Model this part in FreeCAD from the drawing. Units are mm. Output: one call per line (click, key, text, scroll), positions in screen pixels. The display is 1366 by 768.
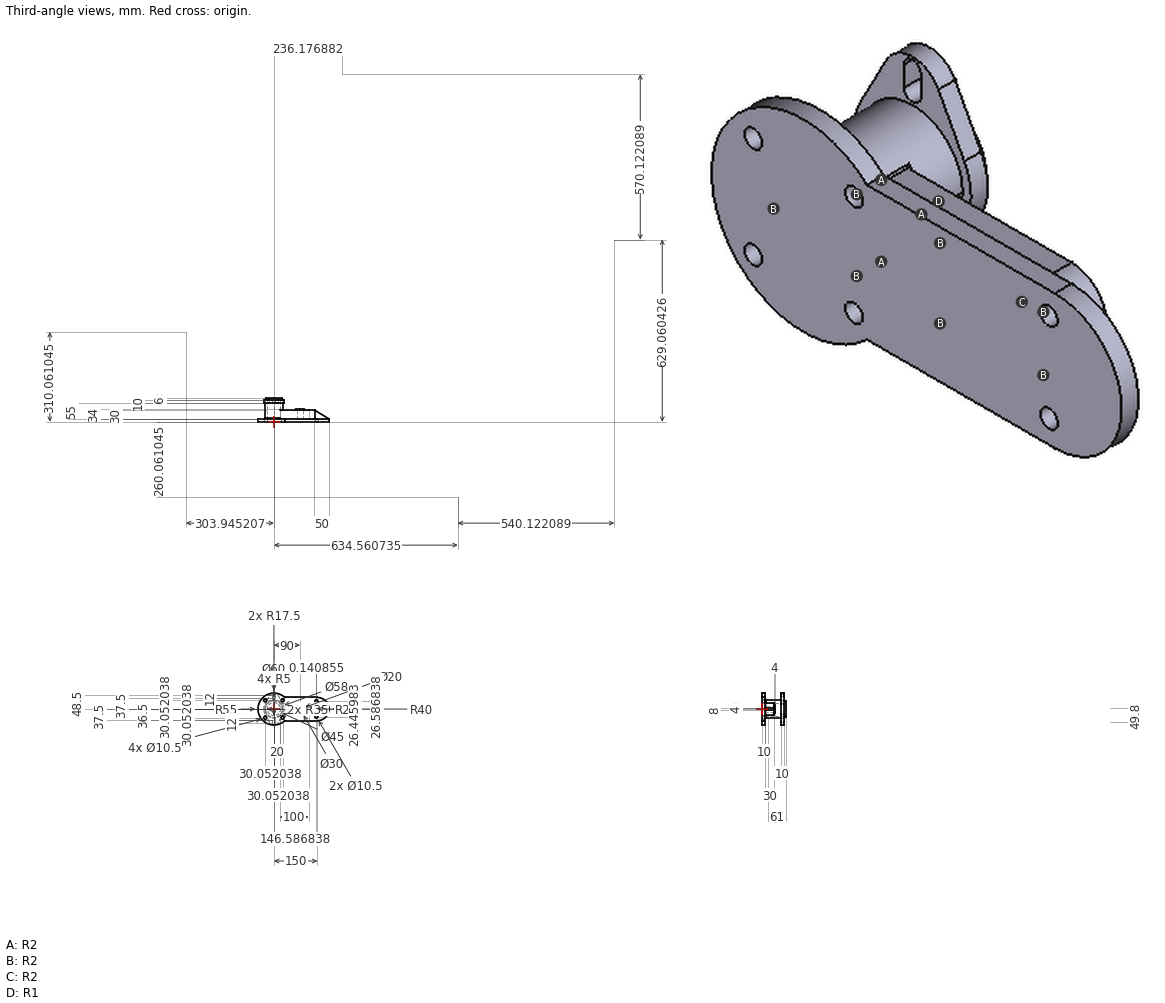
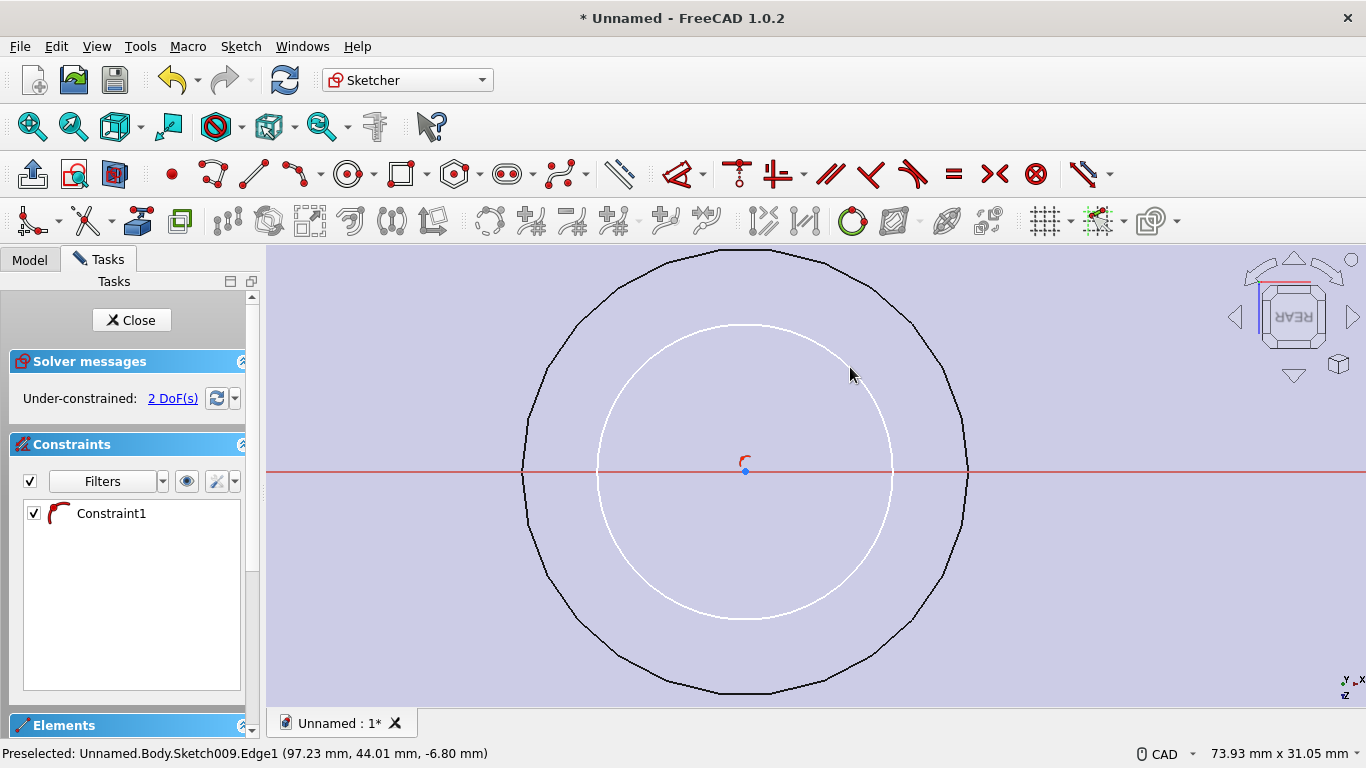
key(d)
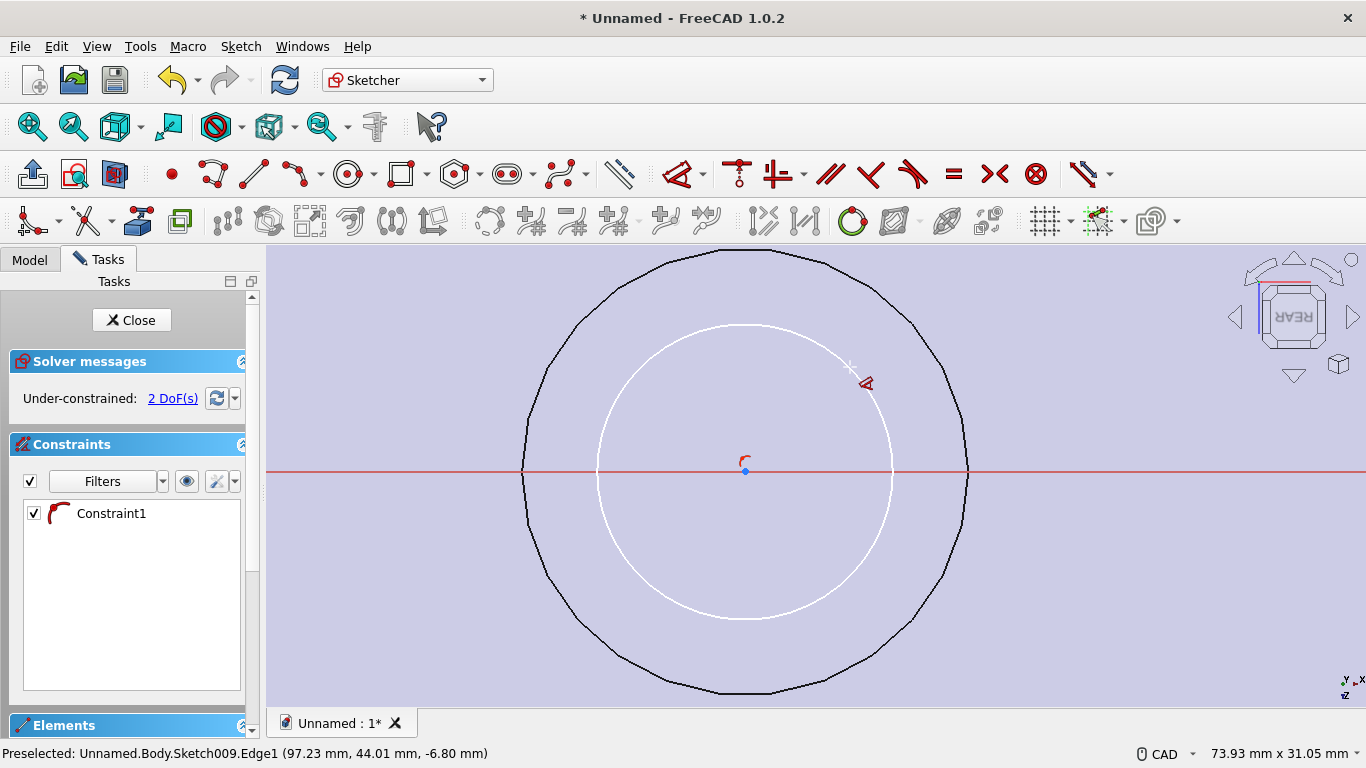
click(849, 367)
click(872, 344)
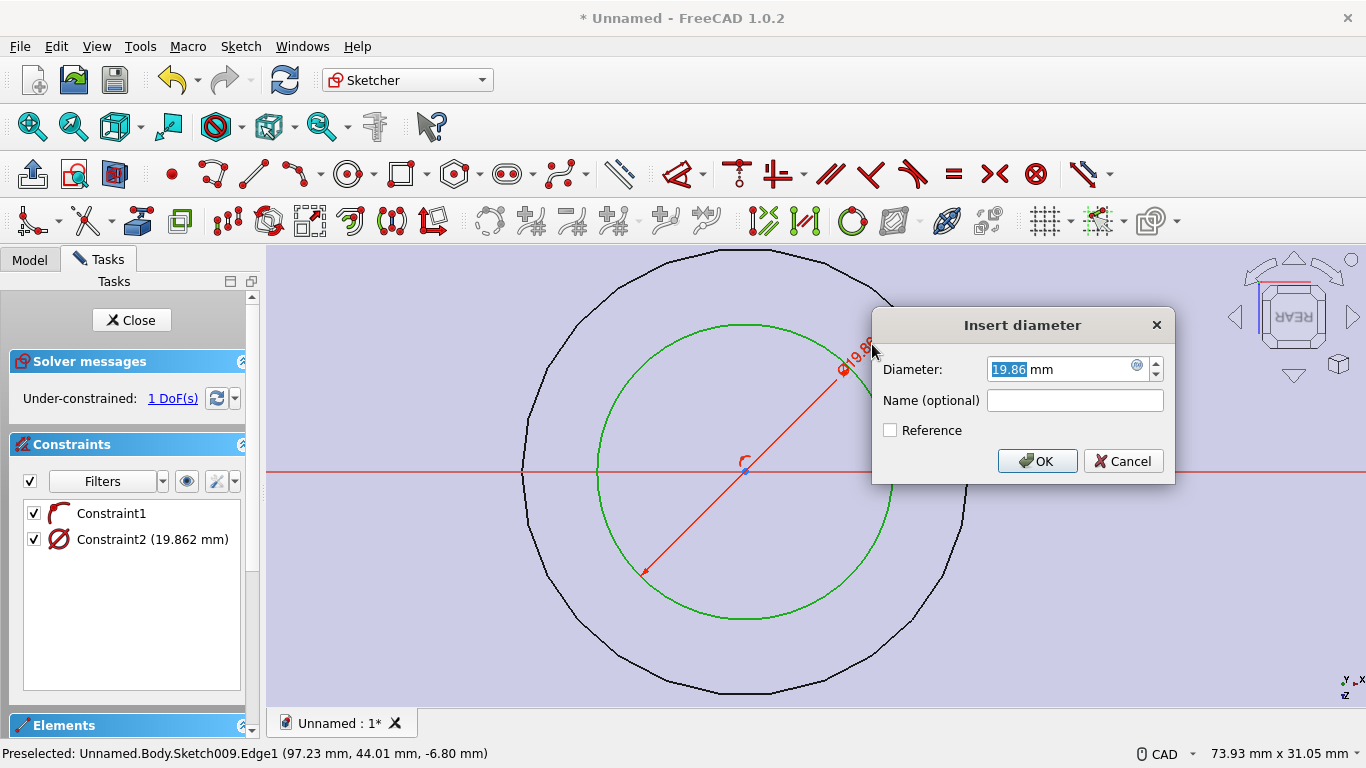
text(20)
key(Return)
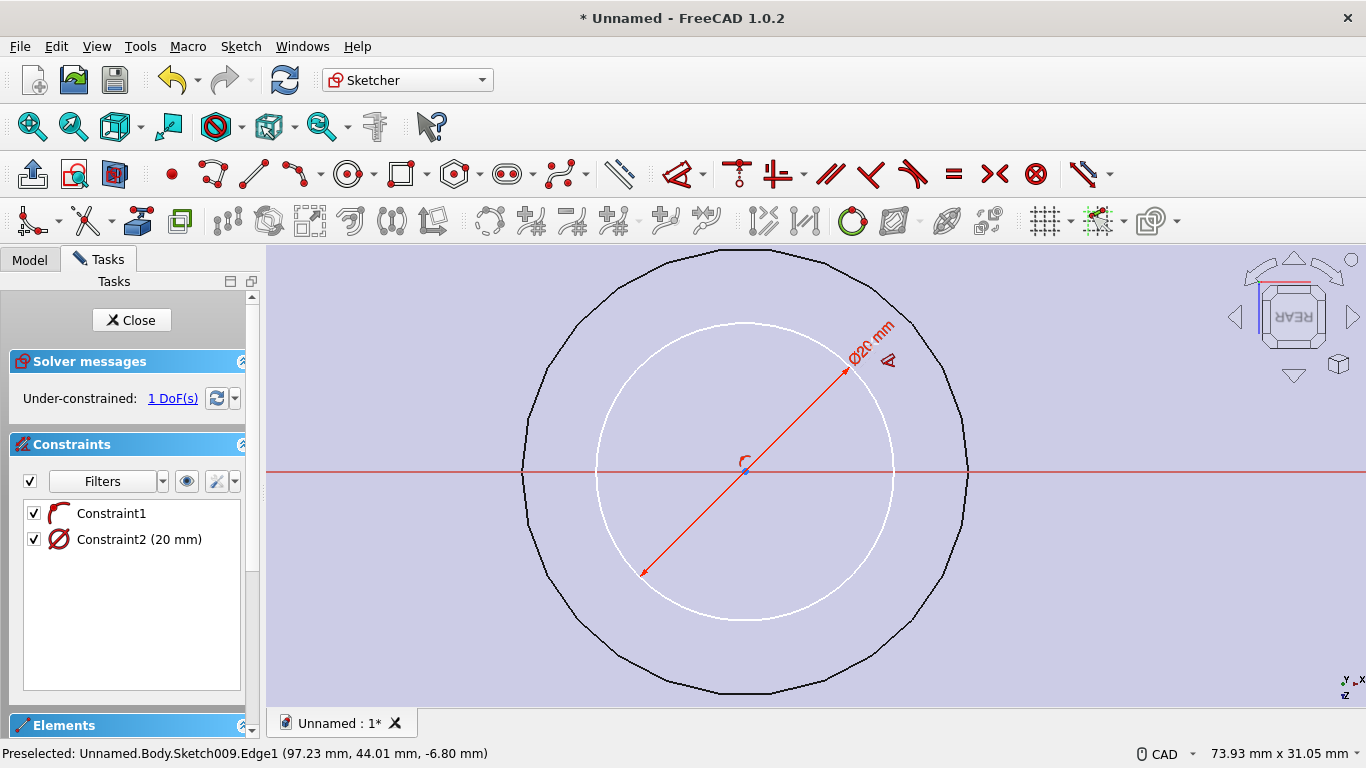
click(745, 472)
click(520, 506)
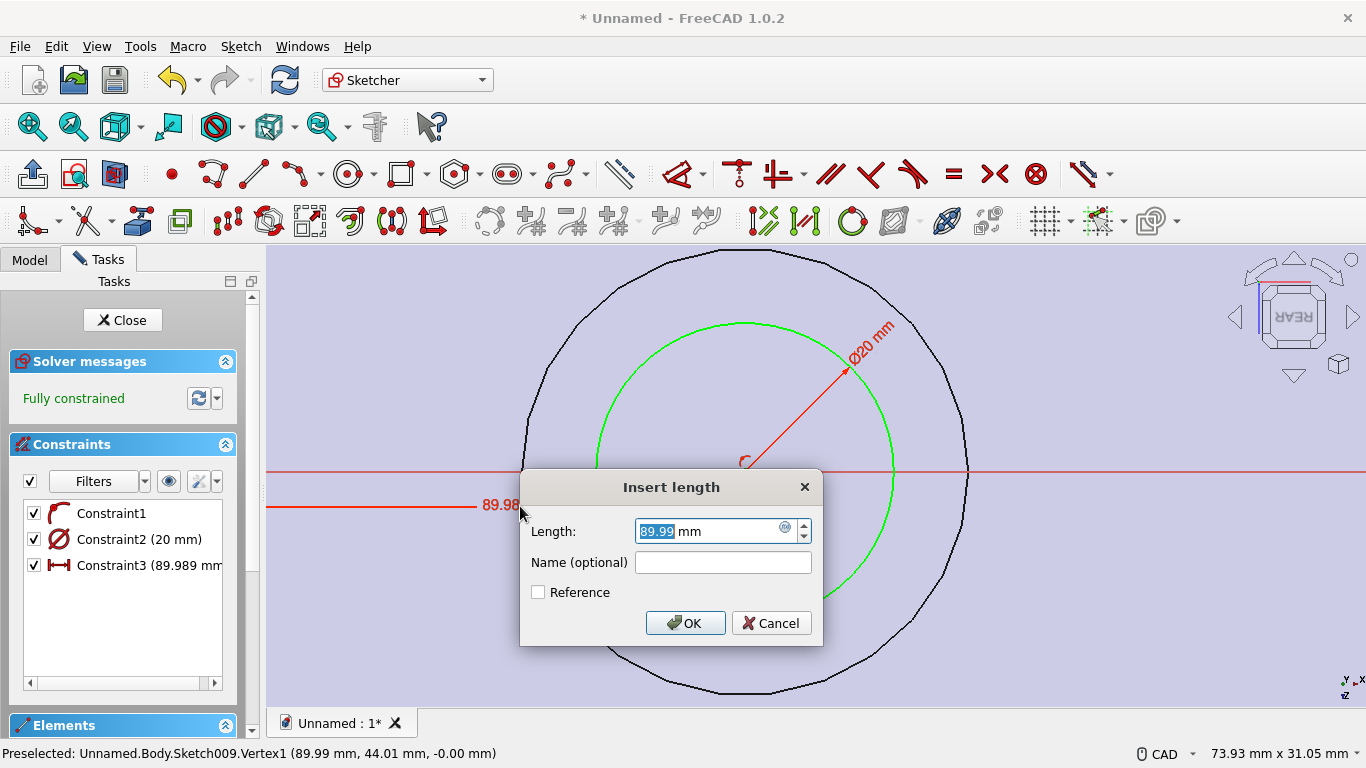
text(90)
key(Return)
key(Escape)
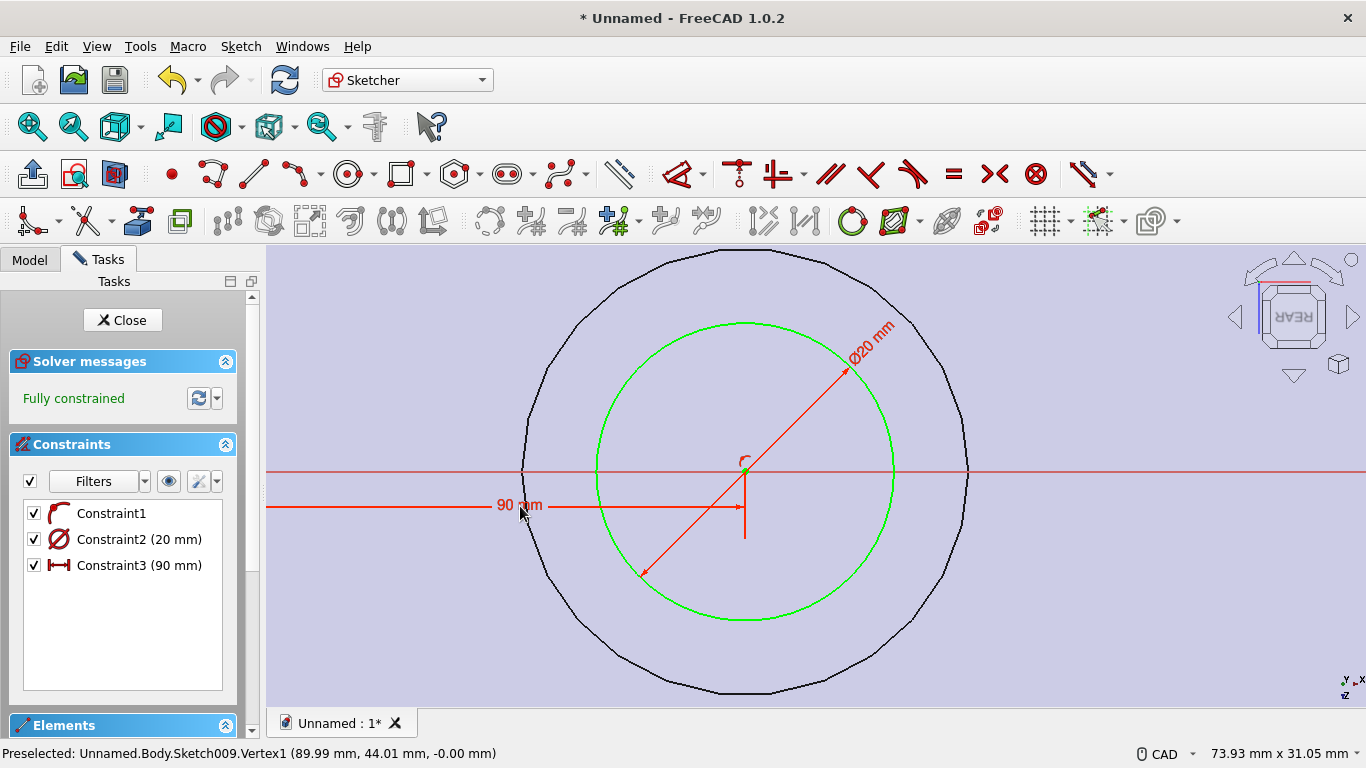
click(123, 320)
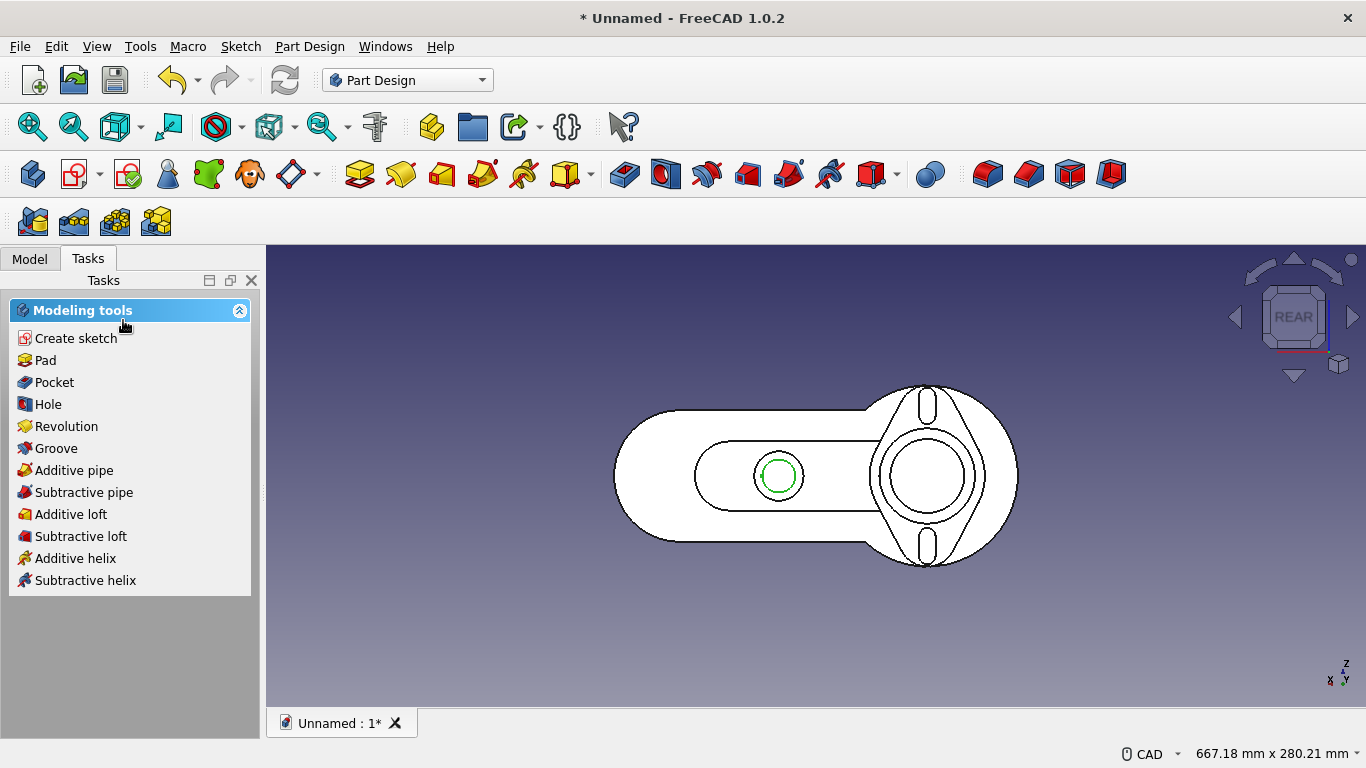
click(625, 174)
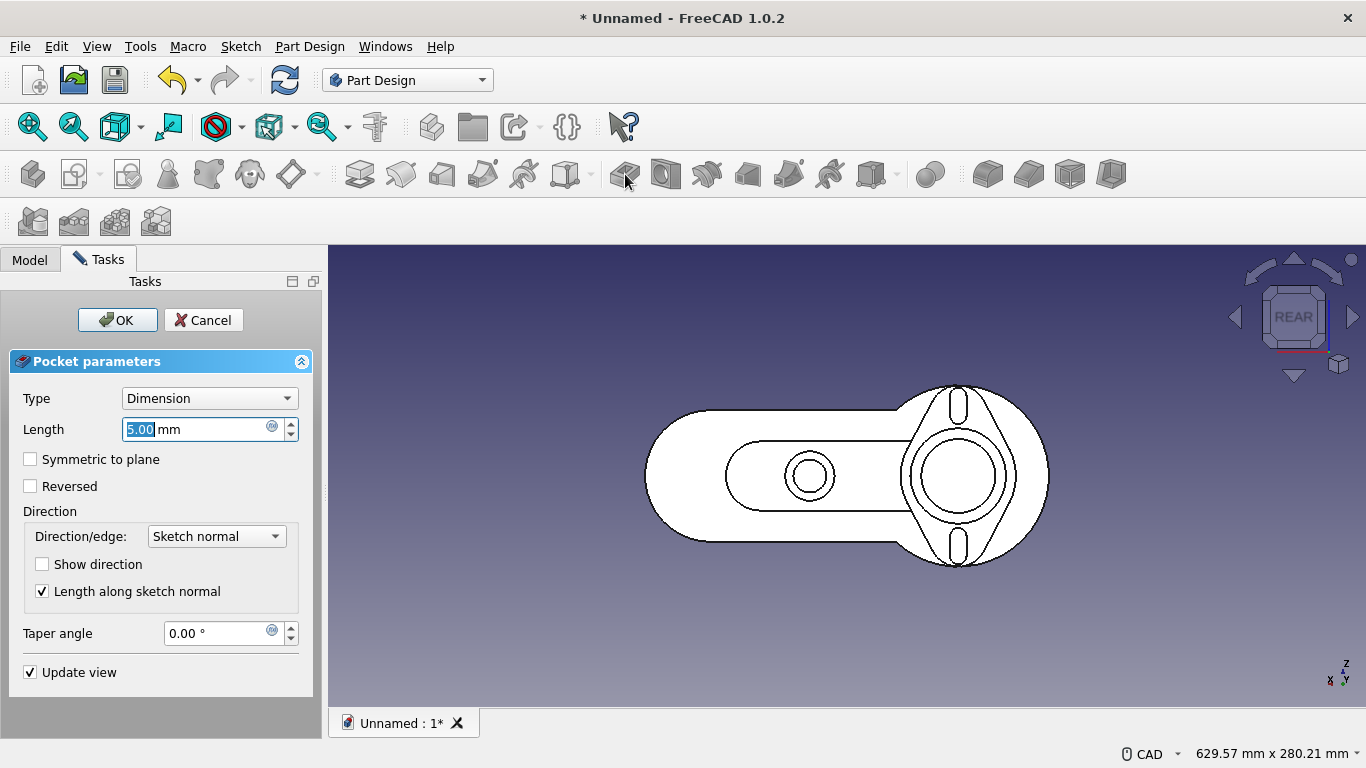
text(34)
key(Tab)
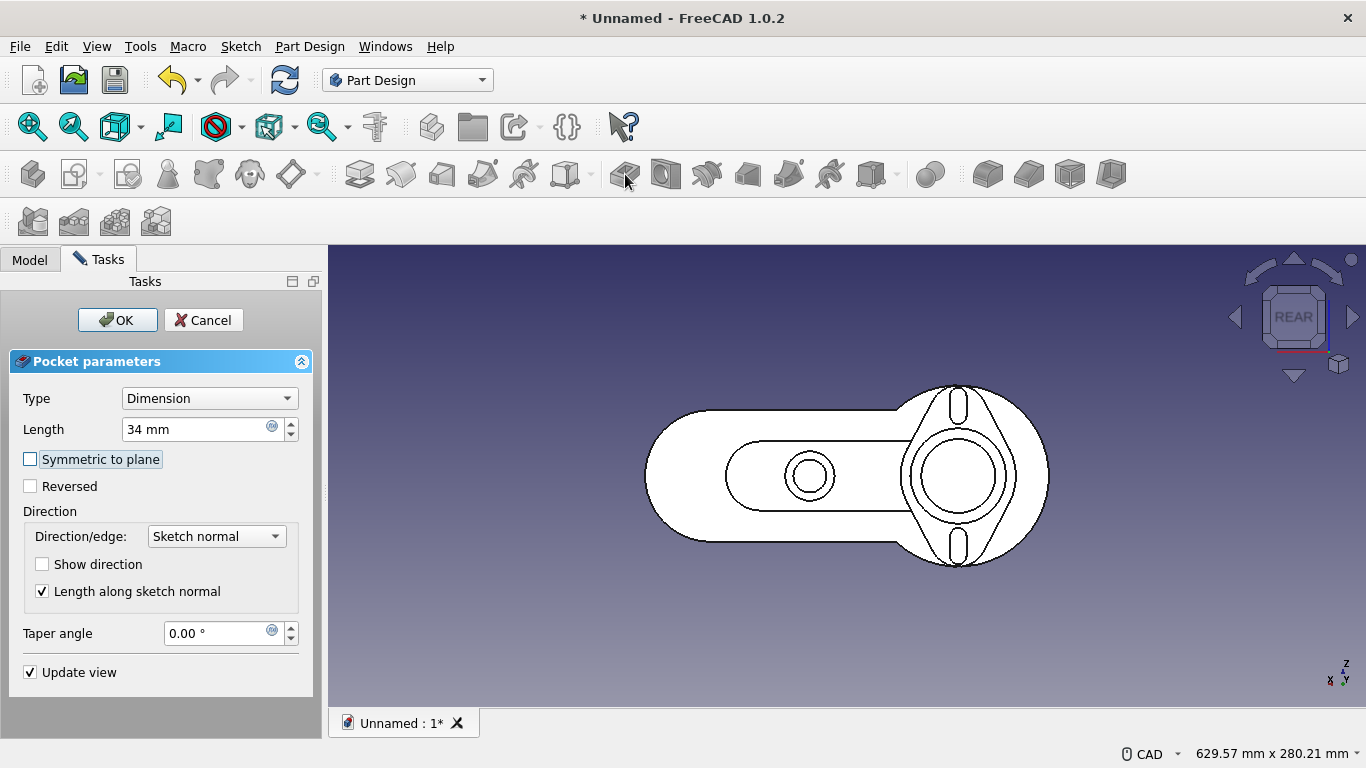
click(118, 320)